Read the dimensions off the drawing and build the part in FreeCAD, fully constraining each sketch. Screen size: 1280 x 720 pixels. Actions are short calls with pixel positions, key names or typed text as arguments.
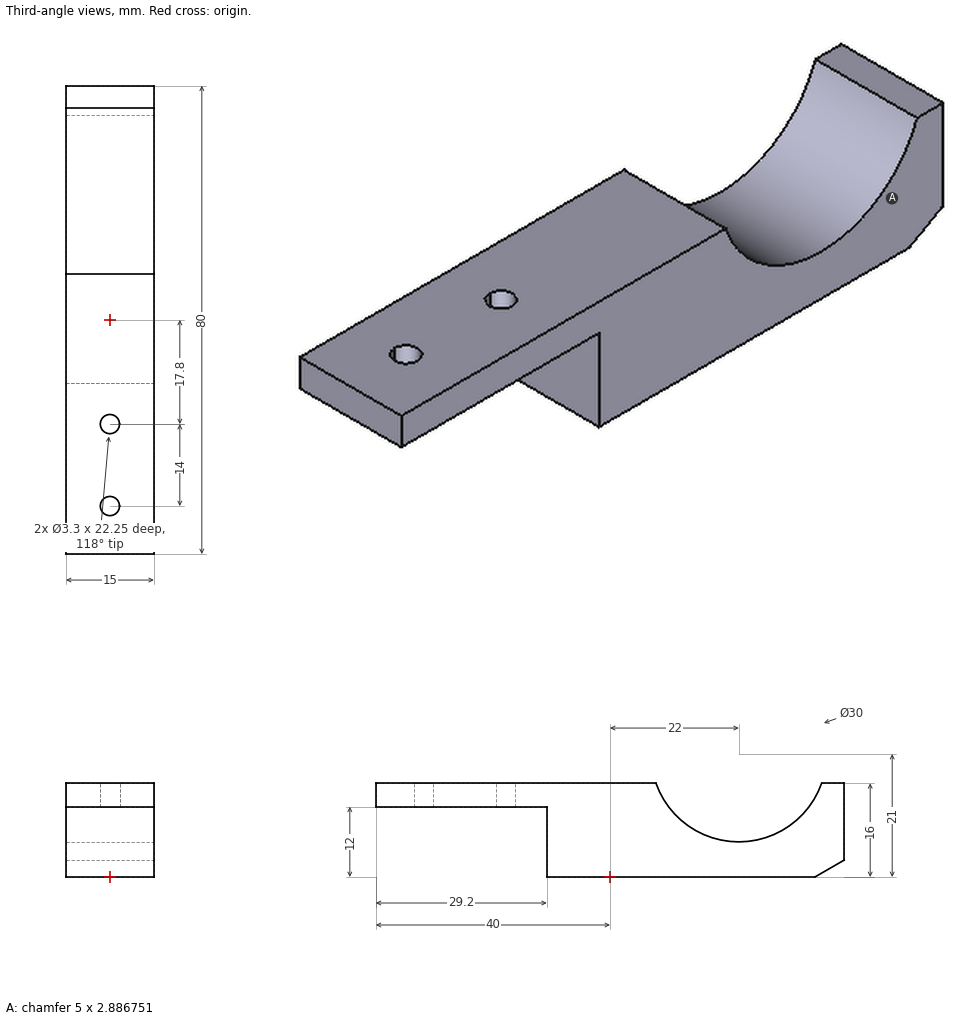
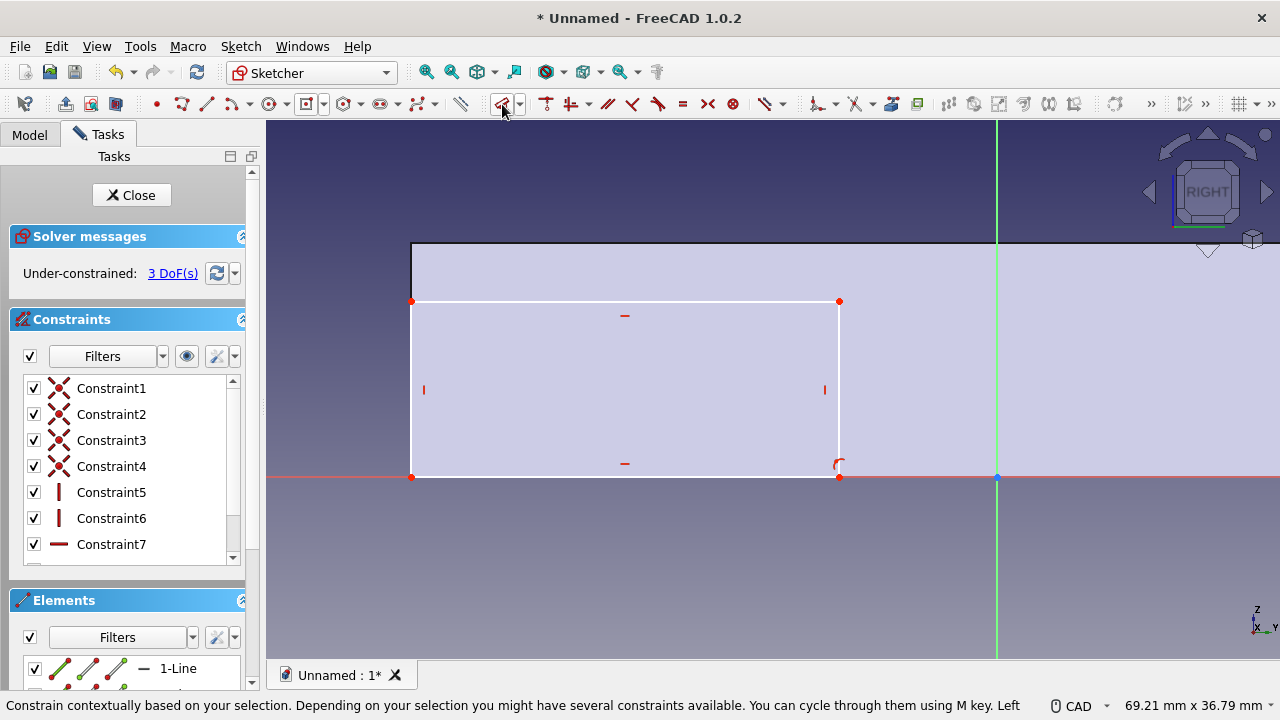
click(411, 355)
click(377, 390)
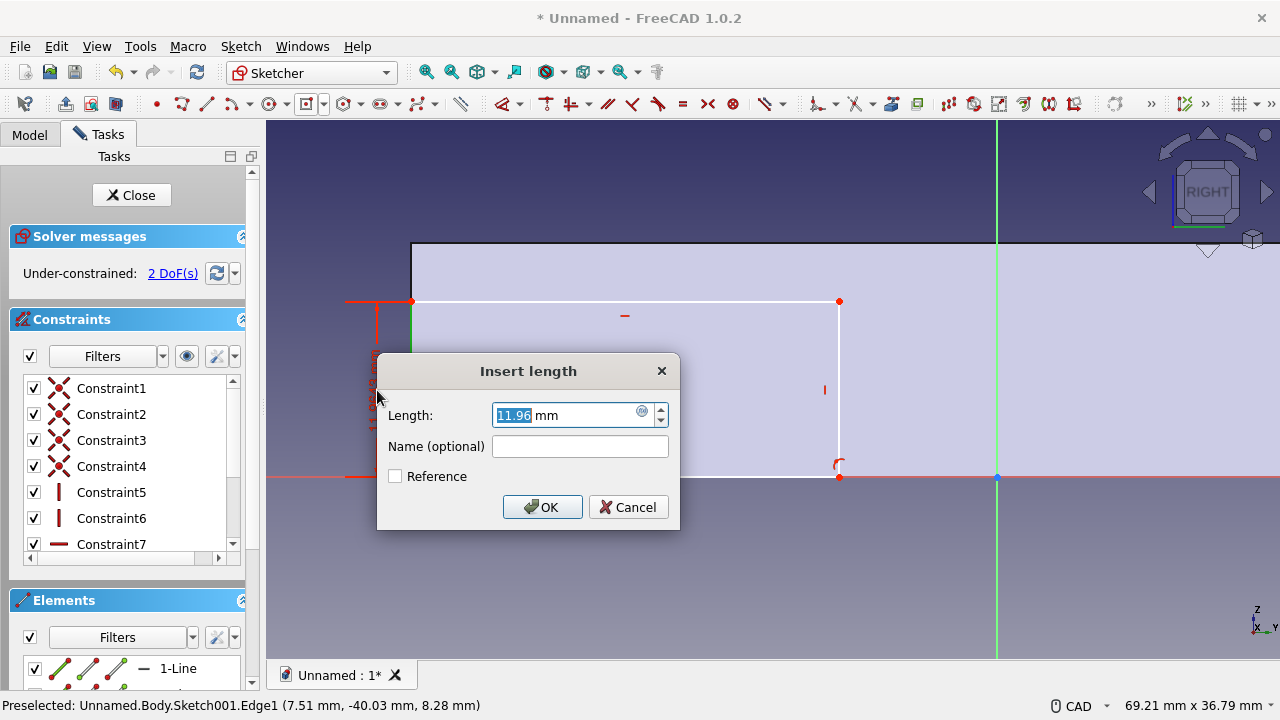
text(12)
key(Return)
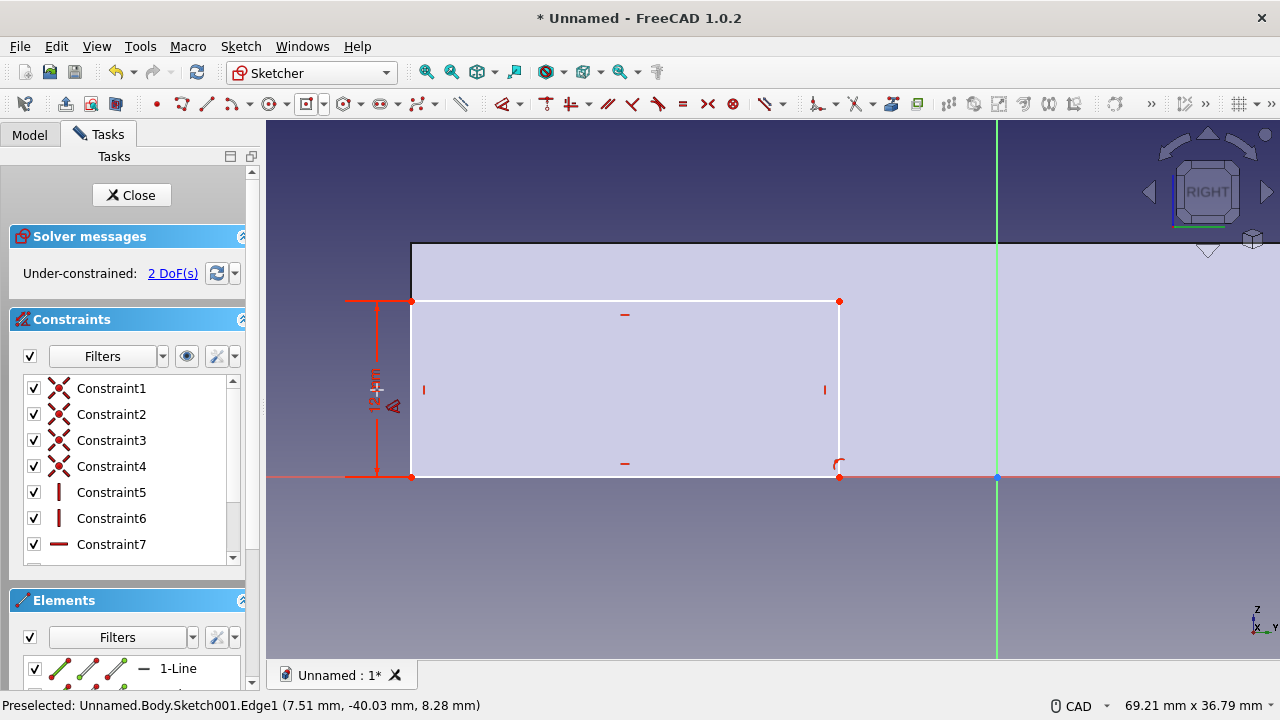
click(411, 301)
click(704, 511)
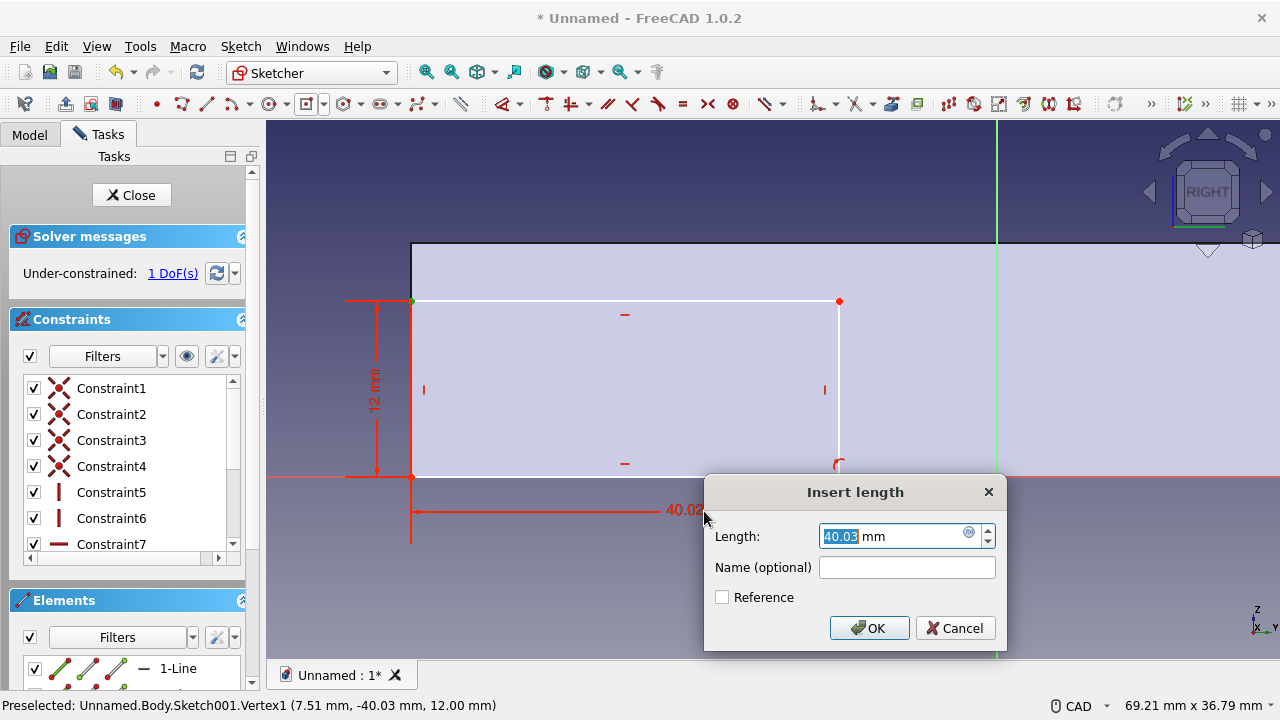
text(40)
key(Return)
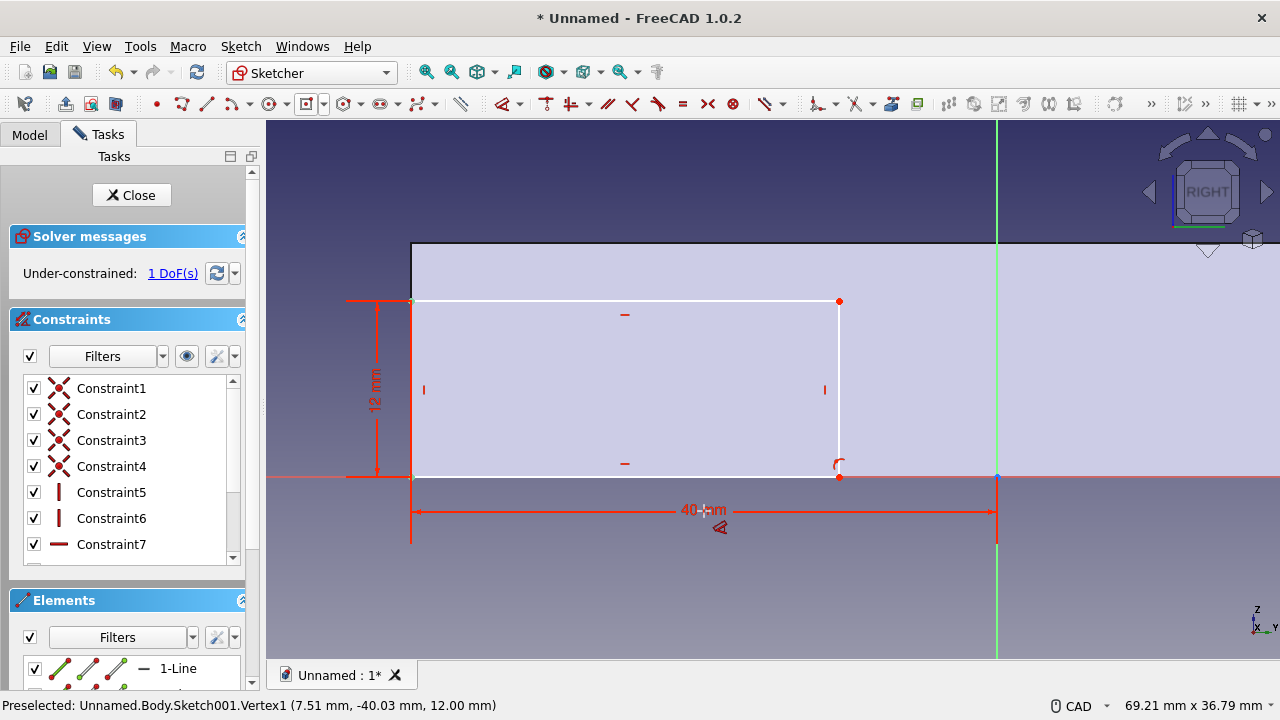
click(540, 477)
click(625, 511)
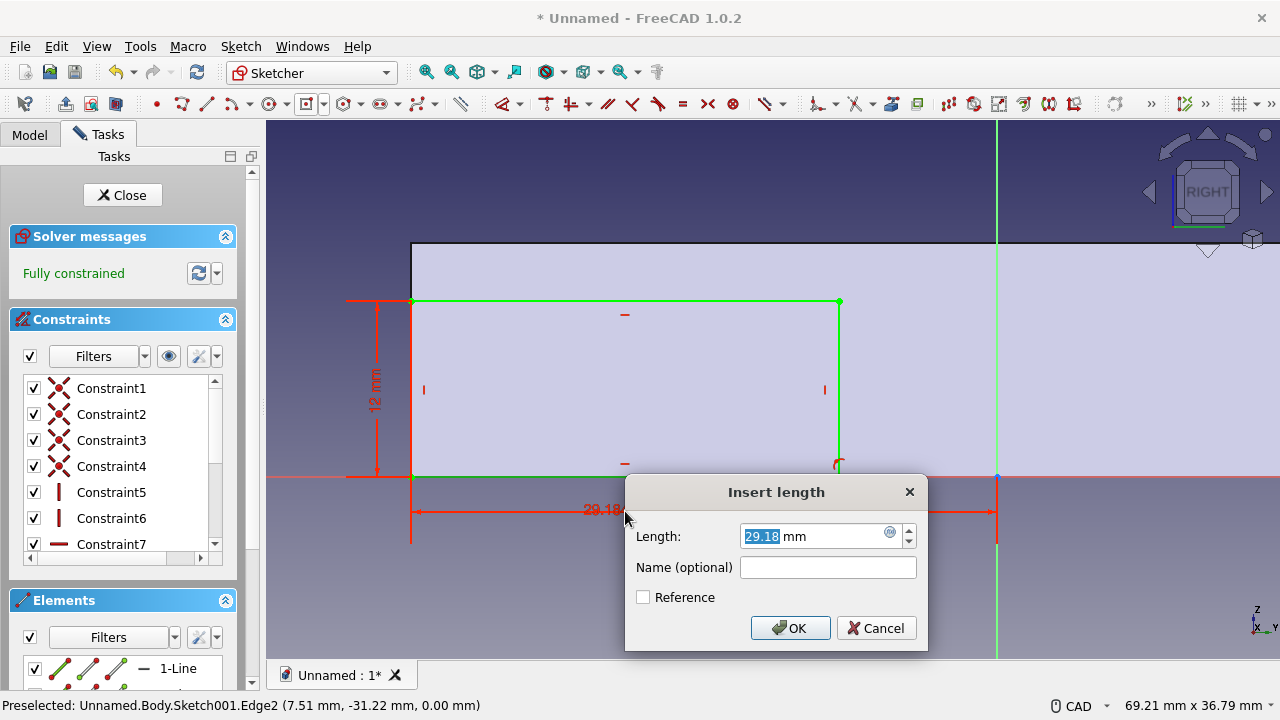
text(29.2)
key(Return)
key(Escape)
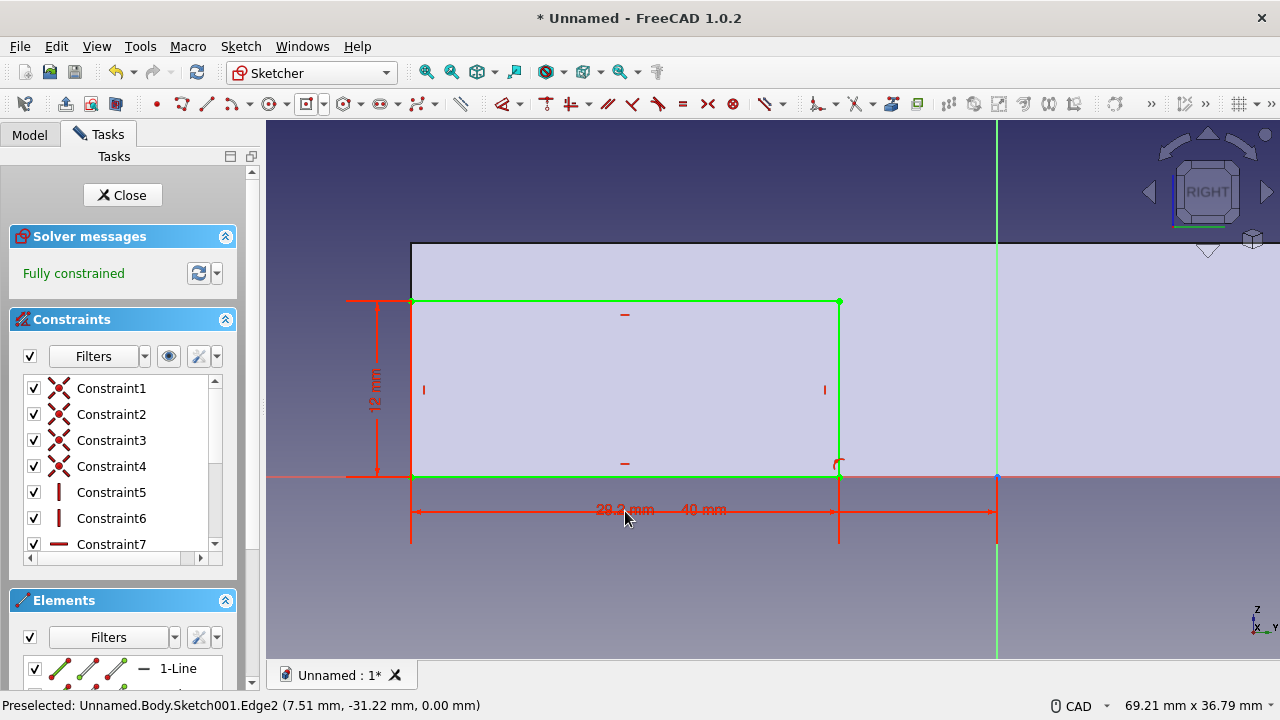
click(123, 195)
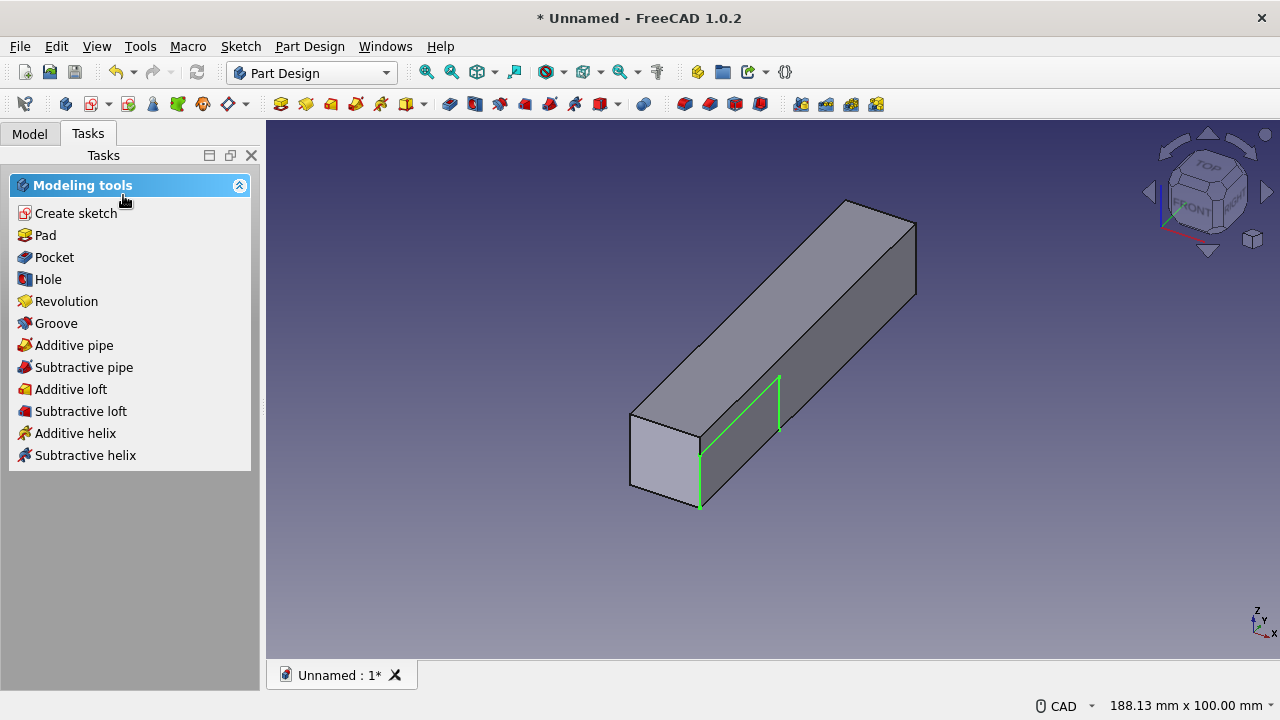
click(450, 104)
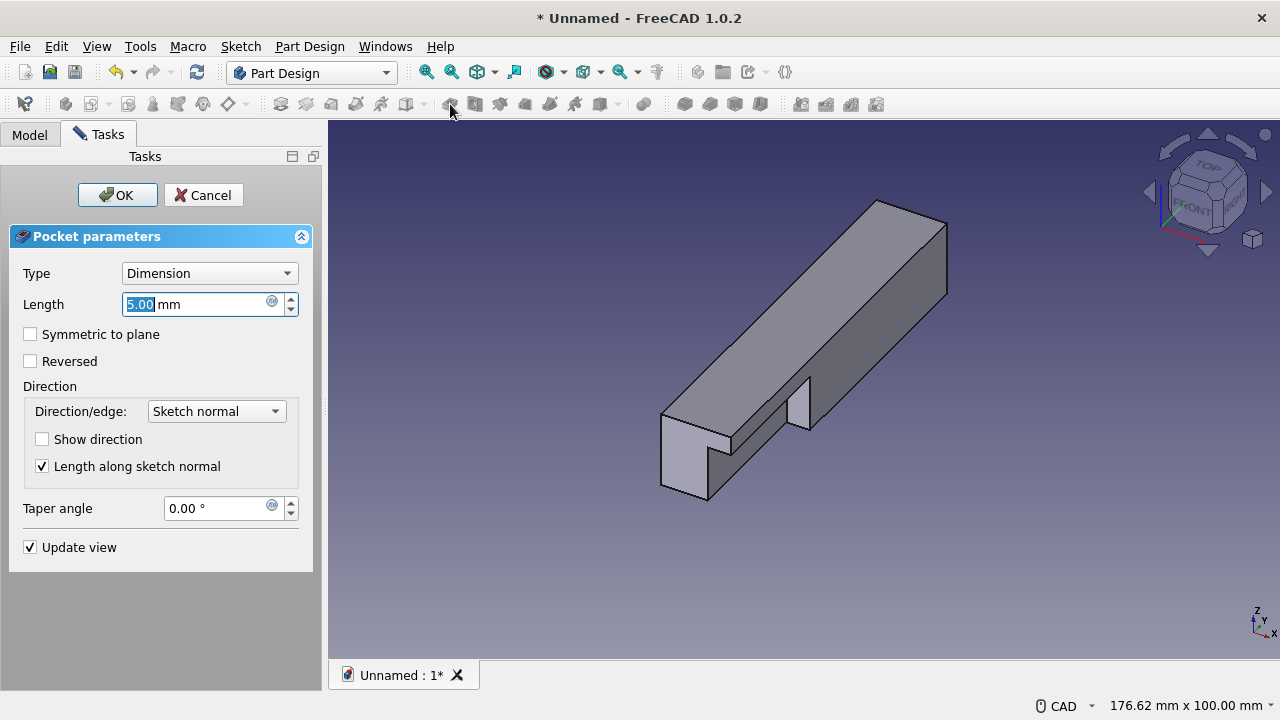
click(210, 274)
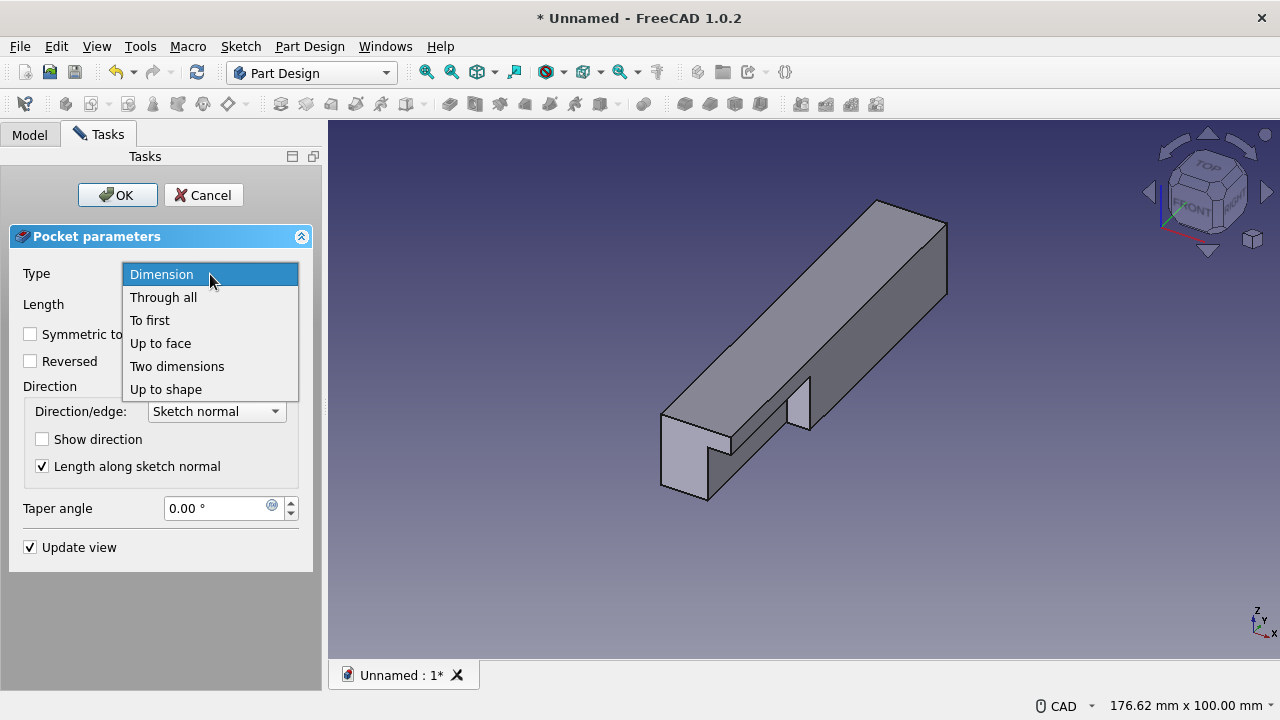
click(208, 298)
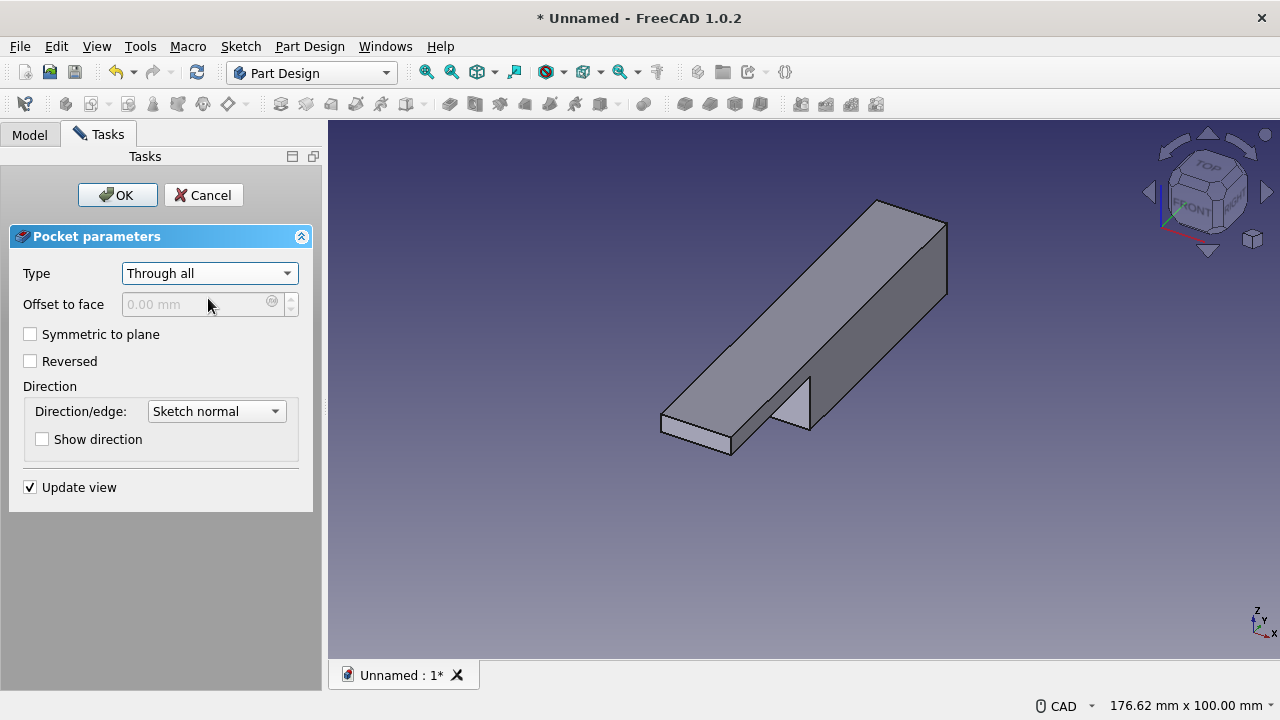
click(118, 195)